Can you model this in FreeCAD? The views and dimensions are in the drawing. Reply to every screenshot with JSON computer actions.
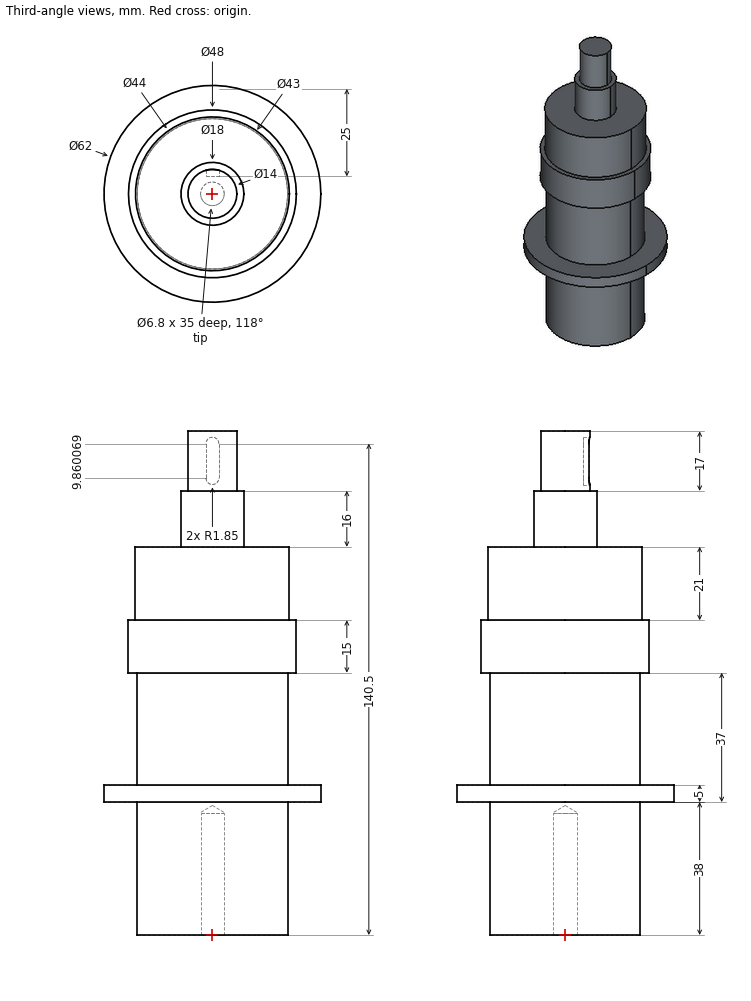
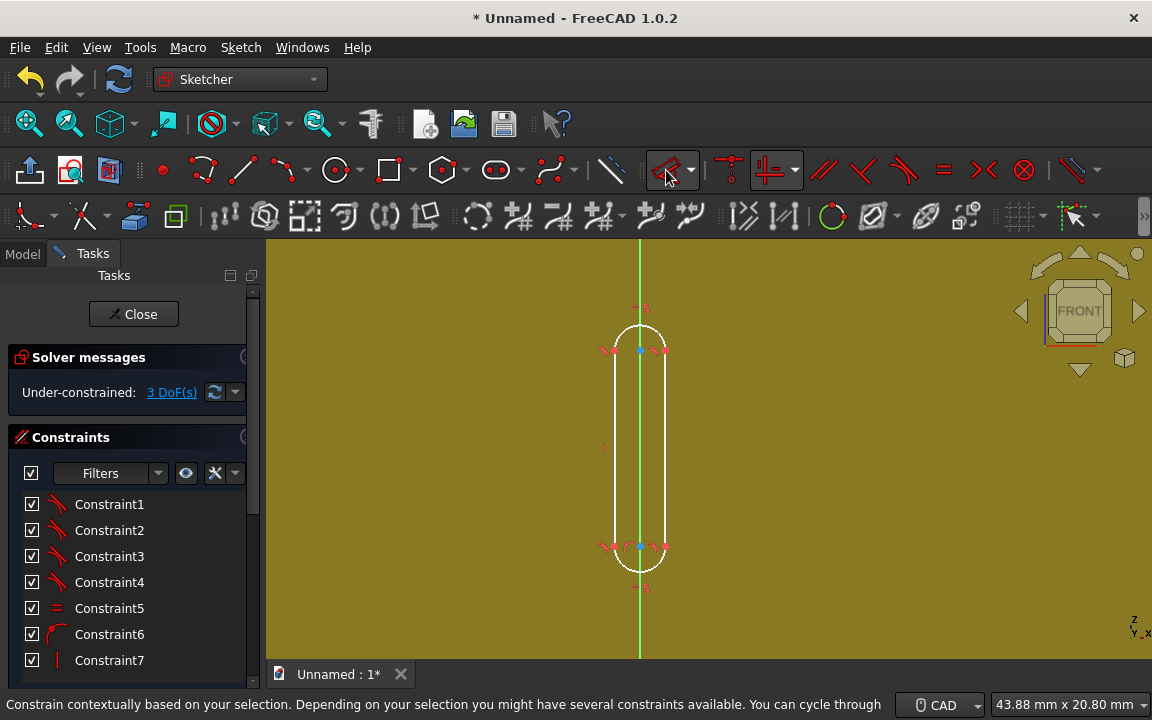
{"action": "left_click", "coordinate": [625, 567]}
{"action": "left_click", "coordinate": [606, 593]}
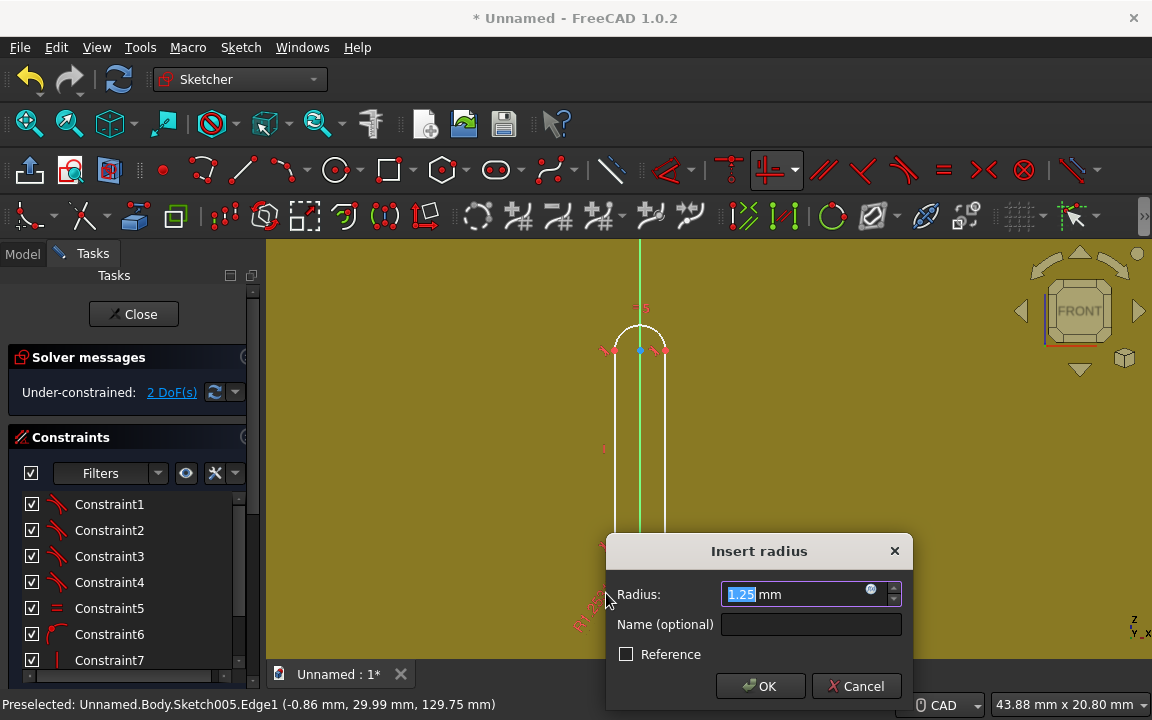
{"action": "type", "text": "1.85"}
{"action": "key", "text": "Return"}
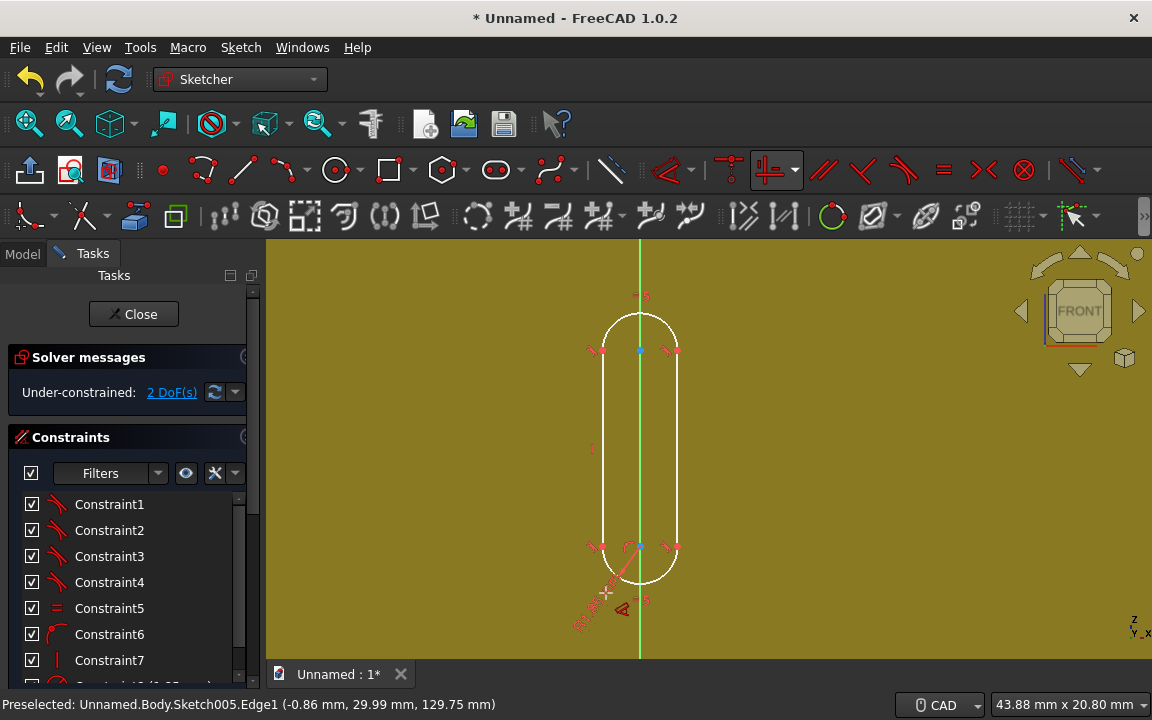
{"action": "left_click", "coordinate": [677, 351]}
{"action": "left_click", "coordinate": [711, 491]}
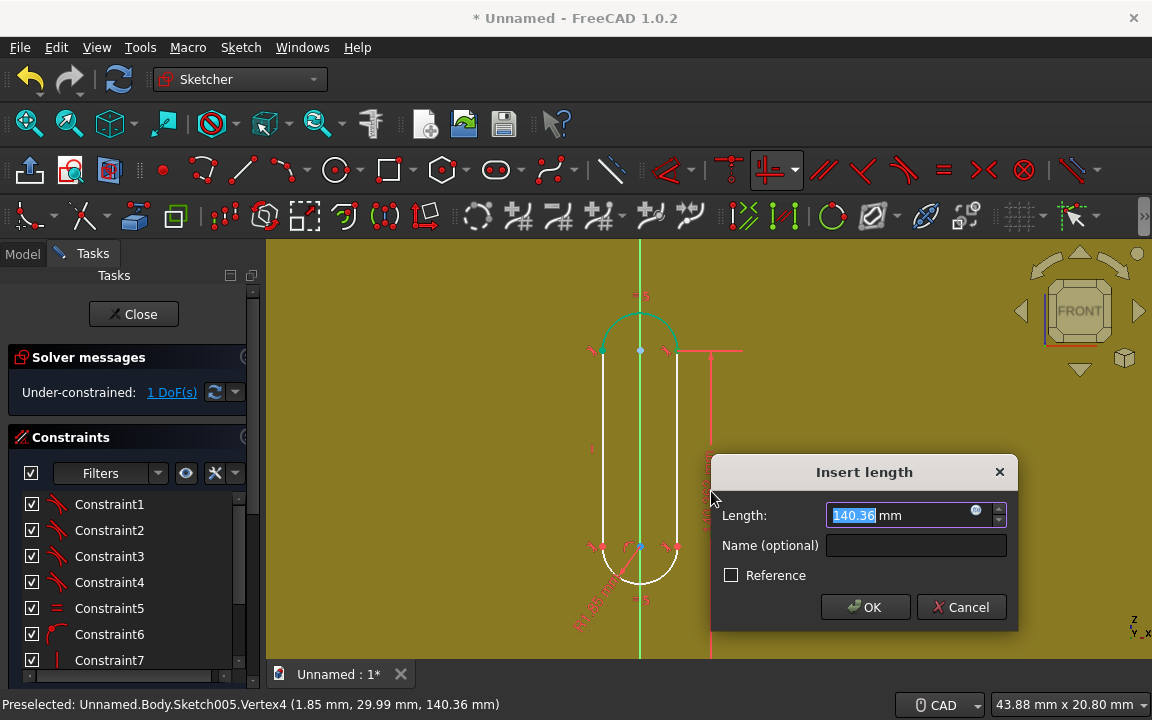
{"action": "type", "text": "140.5"}
{"action": "key", "text": "Return"}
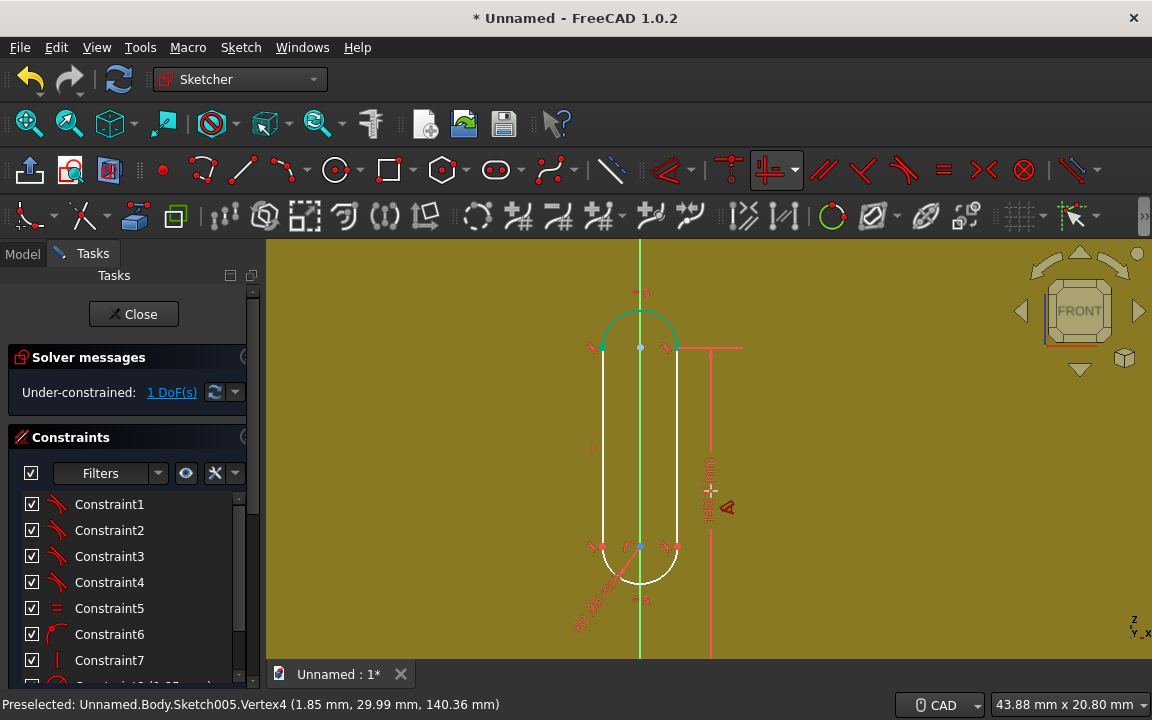
{"action": "left_click", "coordinate": [603, 487]}
{"action": "left_click", "coordinate": [569, 447]}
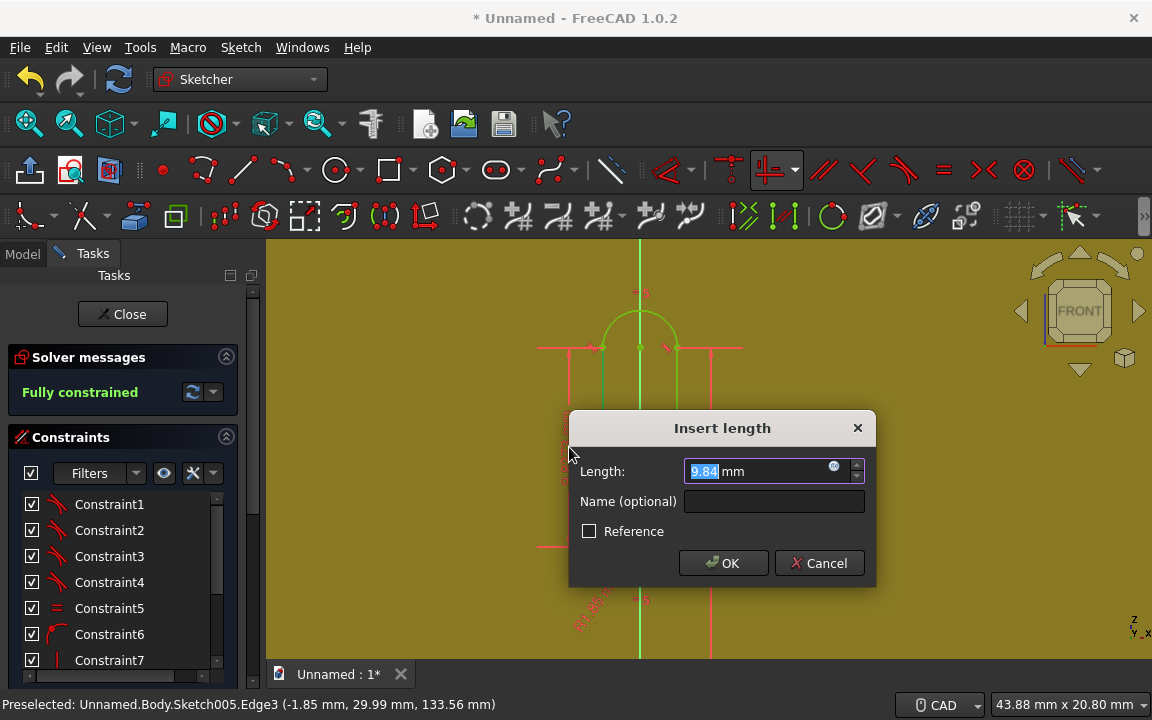
{"action": "type", "text": "9.860069"}
{"action": "key", "text": "Return"}
{"action": "key", "text": "Escape"}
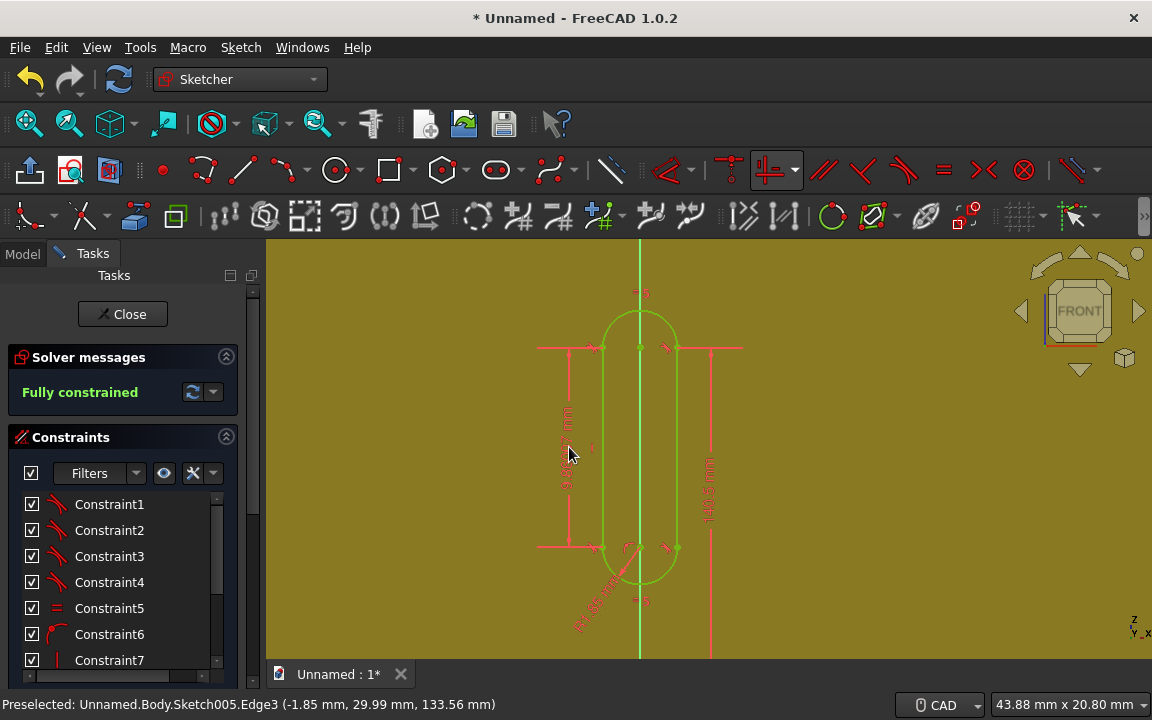
{"action": "left_click", "coordinate": [123, 314]}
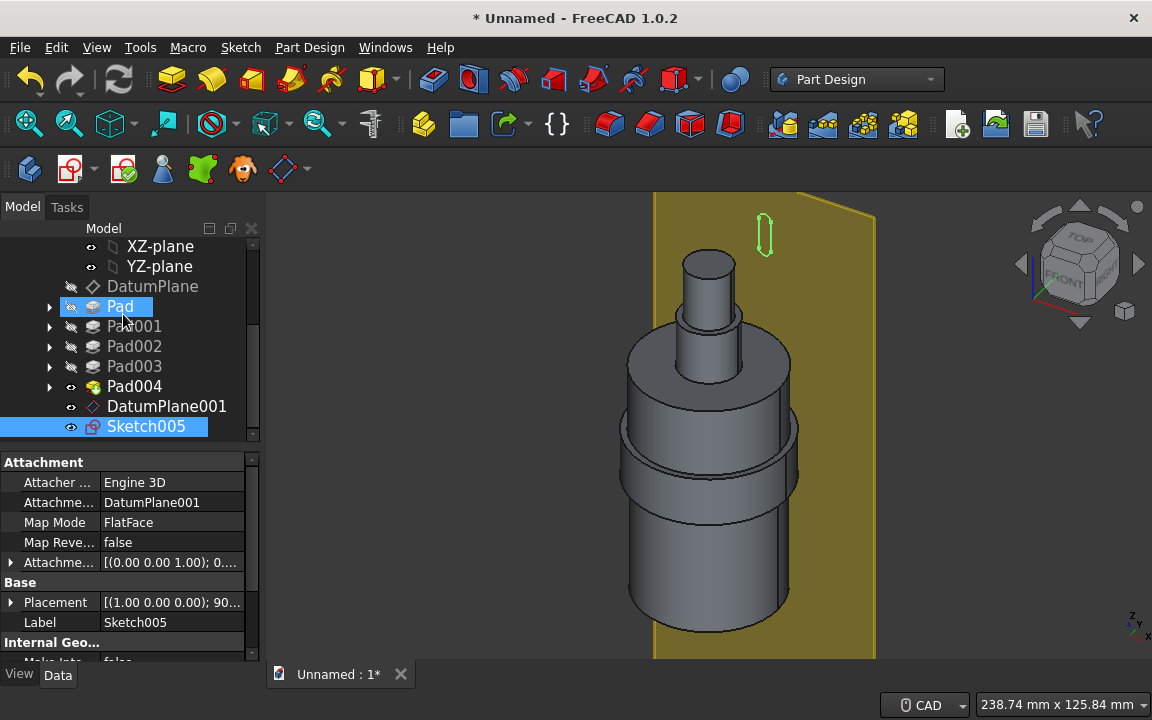
{"action": "left_click", "coordinate": [434, 80]}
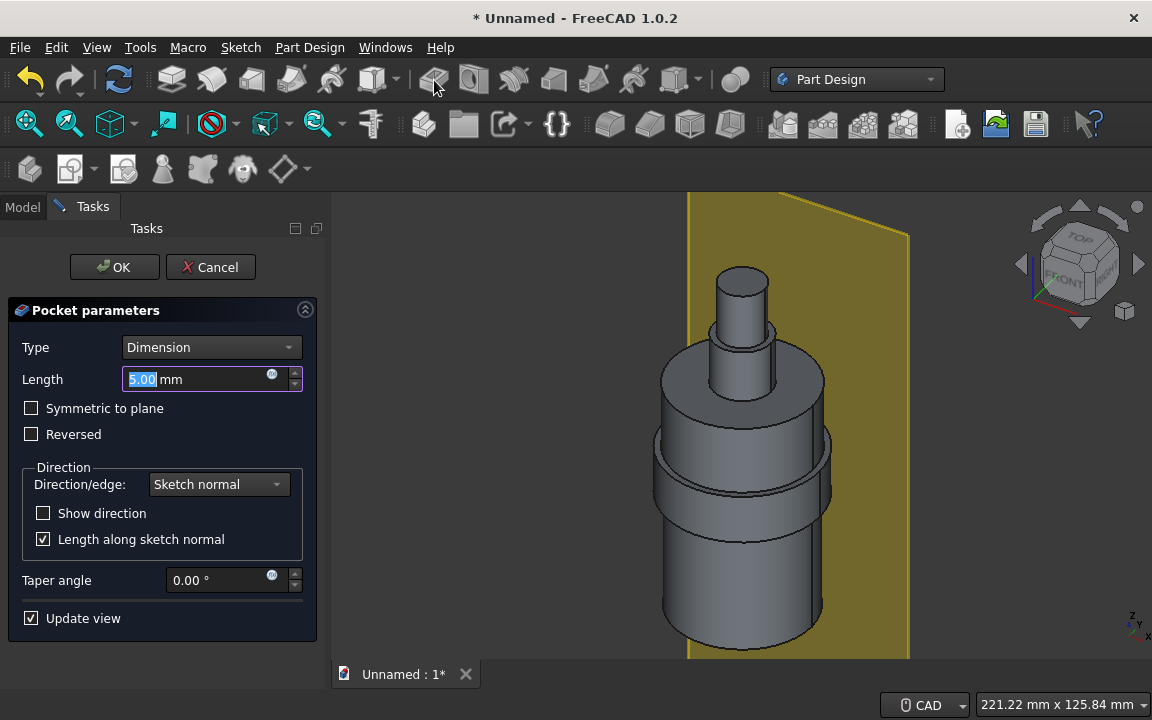
{"action": "type", "text": "25"}
{"action": "key", "text": "Tab"}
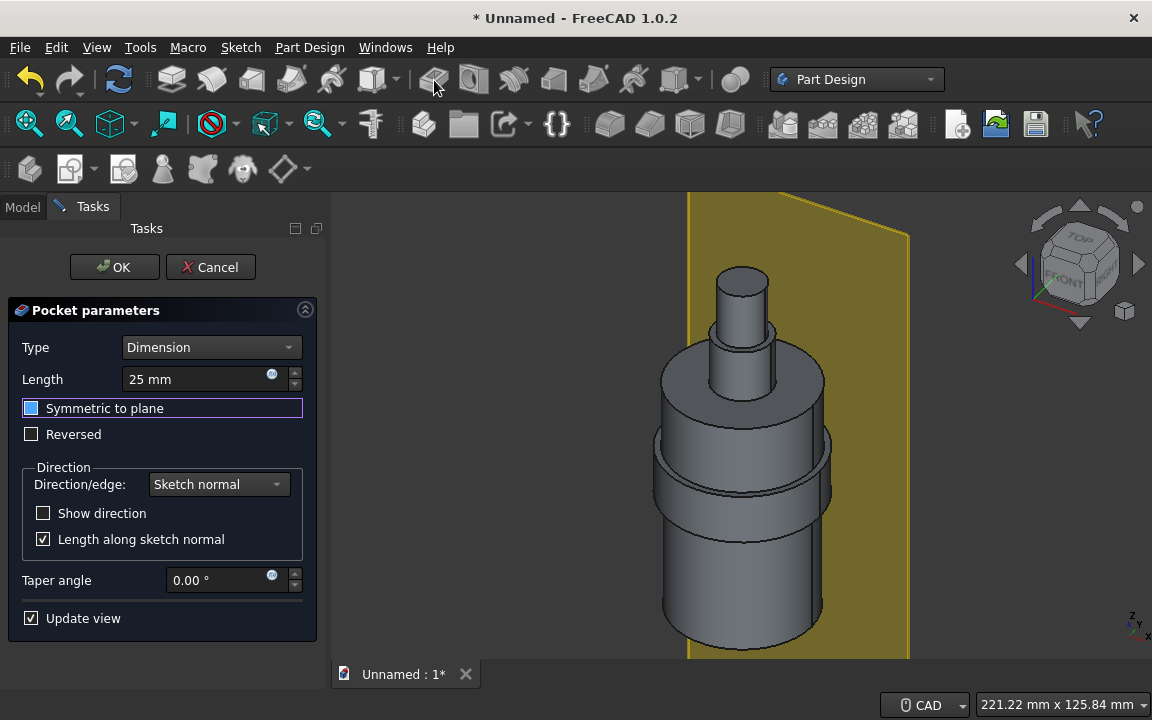
{"action": "left_click", "coordinate": [30, 434]}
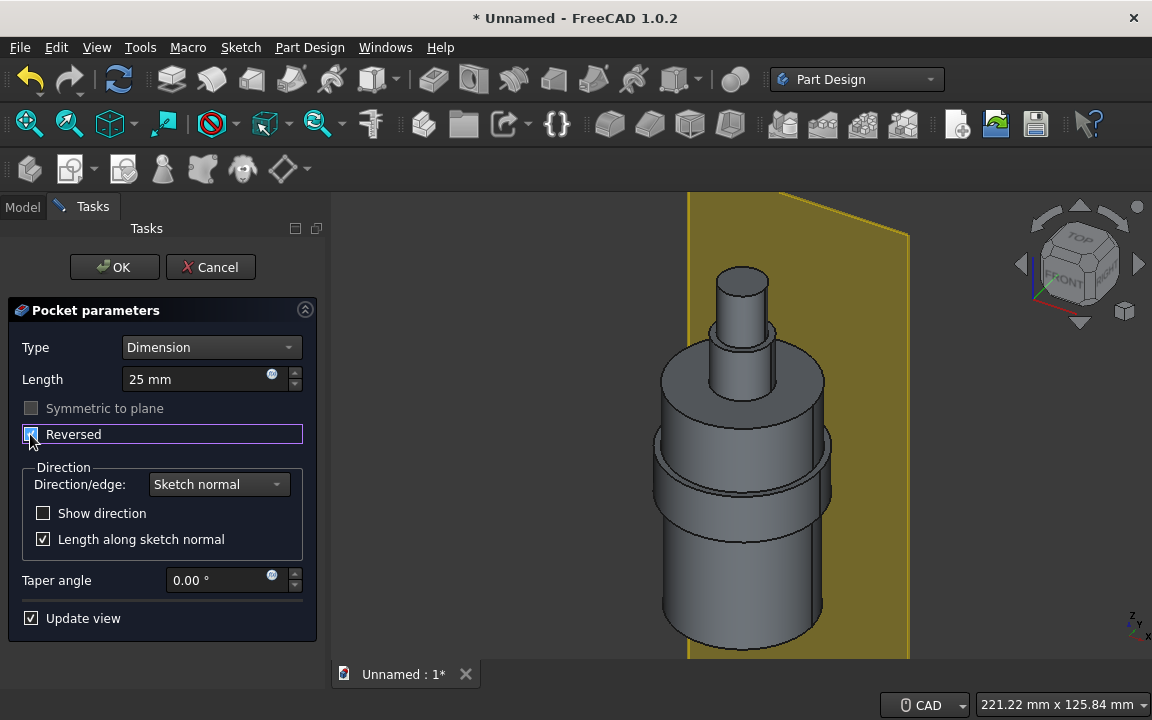
{"action": "left_click", "coordinate": [115, 267]}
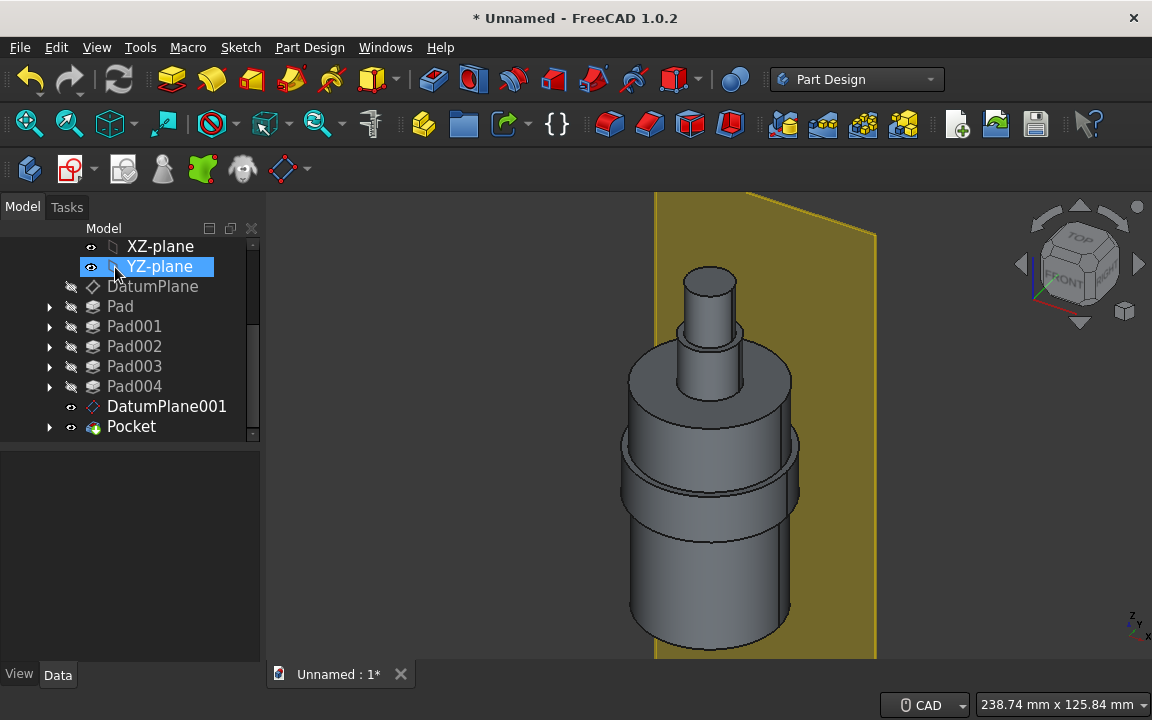
{"action": "left_click", "coordinate": [116, 407]}
{"action": "key", "text": "space"}